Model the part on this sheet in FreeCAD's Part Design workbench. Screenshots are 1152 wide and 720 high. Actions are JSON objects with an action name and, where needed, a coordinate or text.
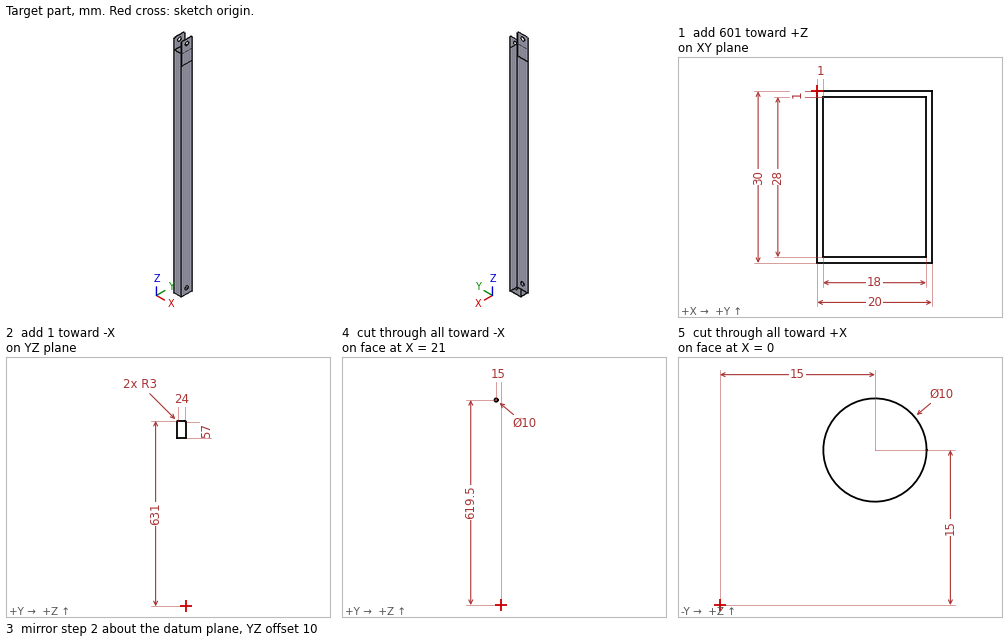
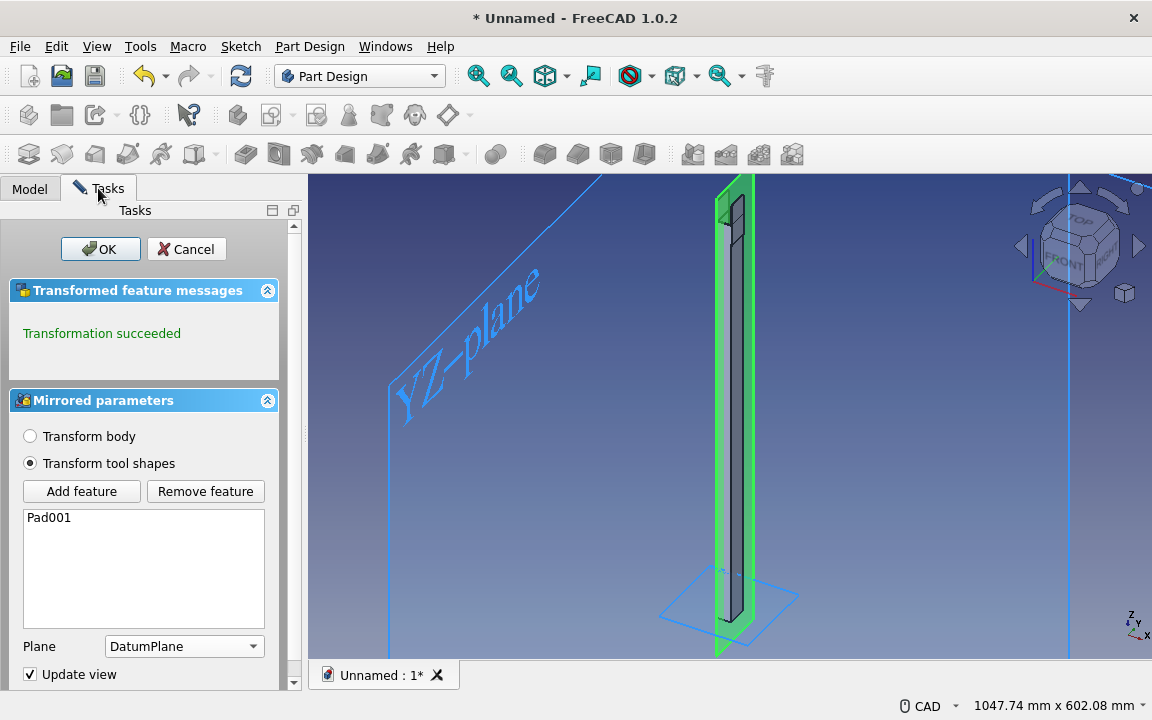
{"action": "left_click", "coordinate": [101, 249]}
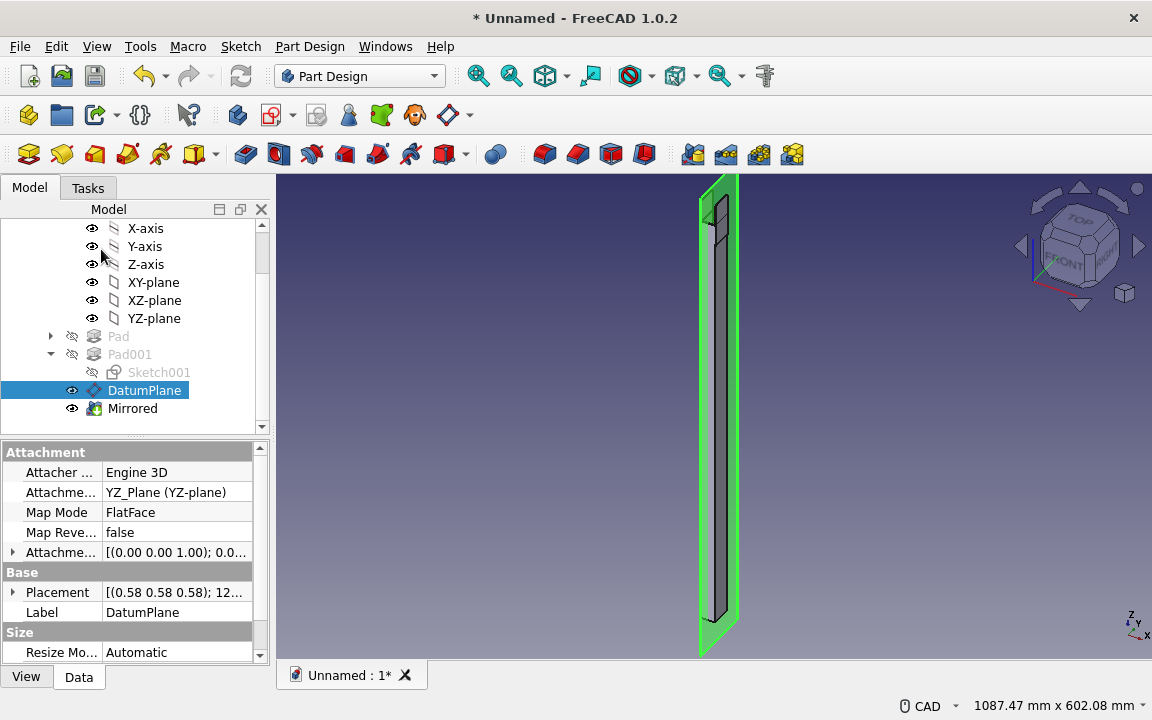
{"action": "left_click", "coordinate": [117, 390]}
{"action": "key", "text": "space"}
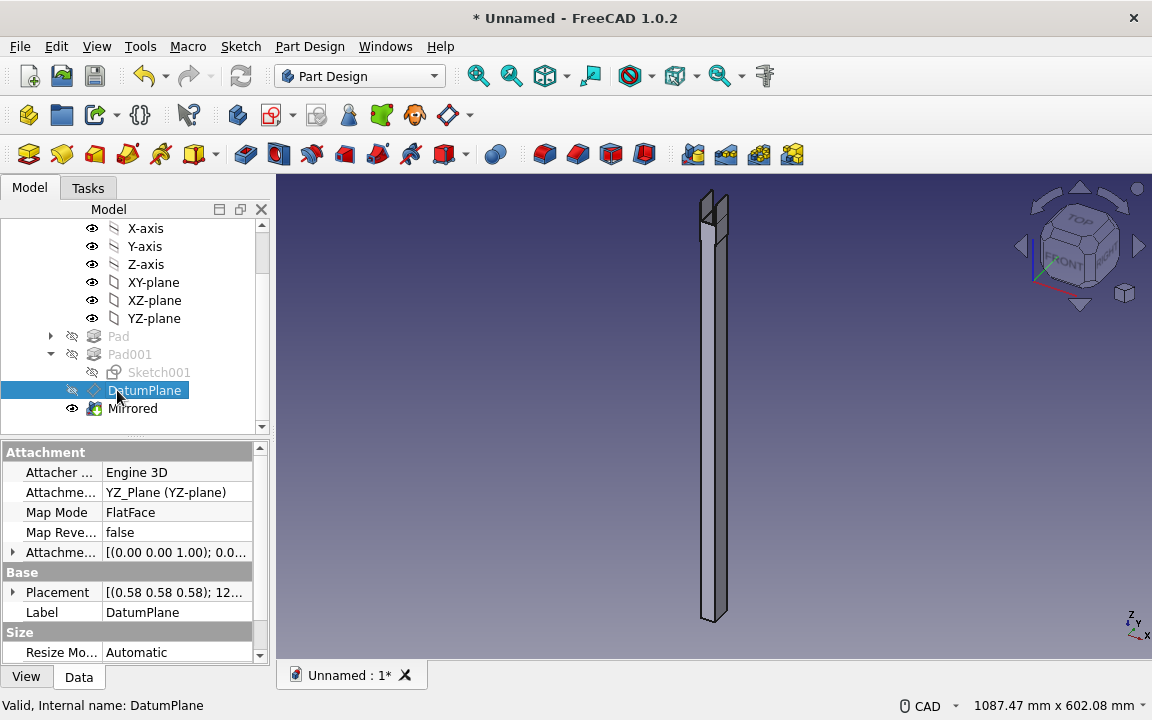
{"action": "key", "text": "0"}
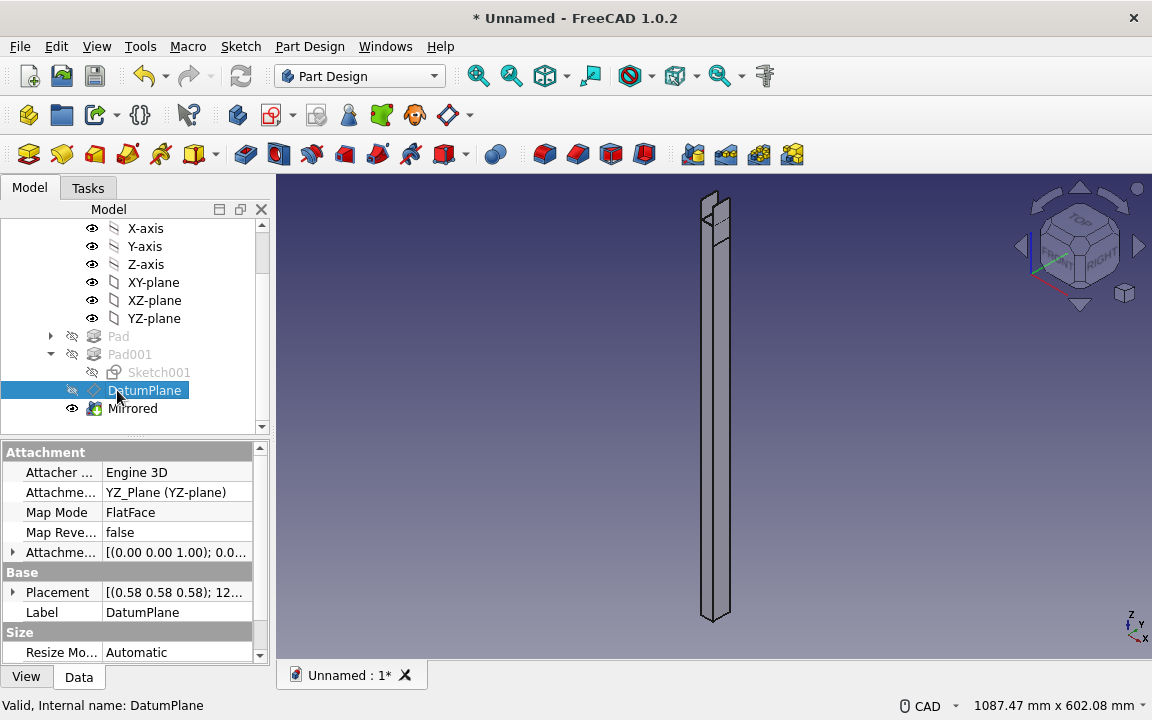
{"action": "left_click", "coordinate": [722, 215]}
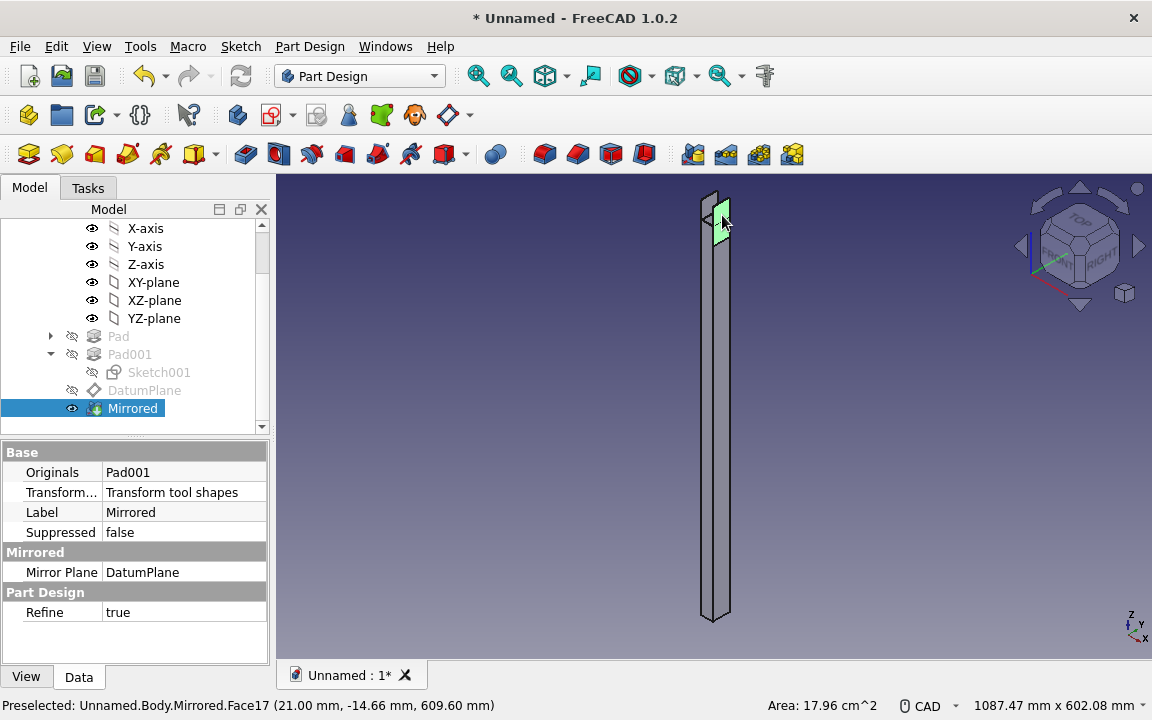
{"action": "left_click", "coordinate": [270, 116]}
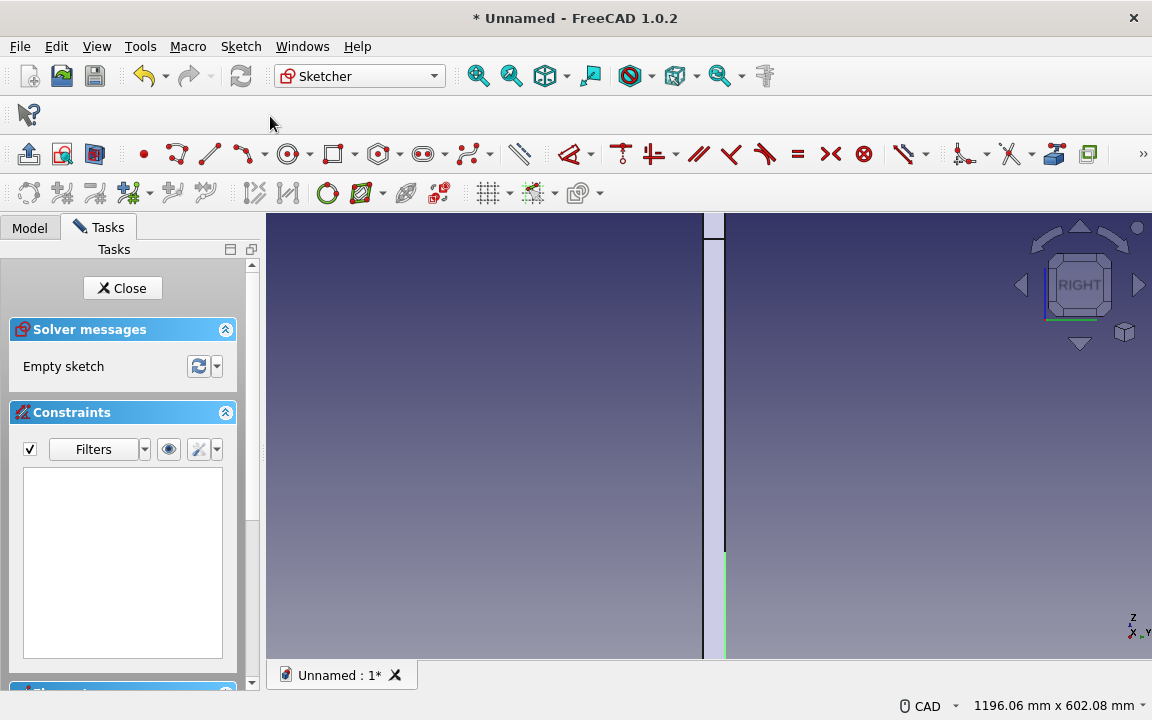
{"action": "scroll", "coordinate": [640, 436], "scroll_direction": "down", "scroll_amount": 5}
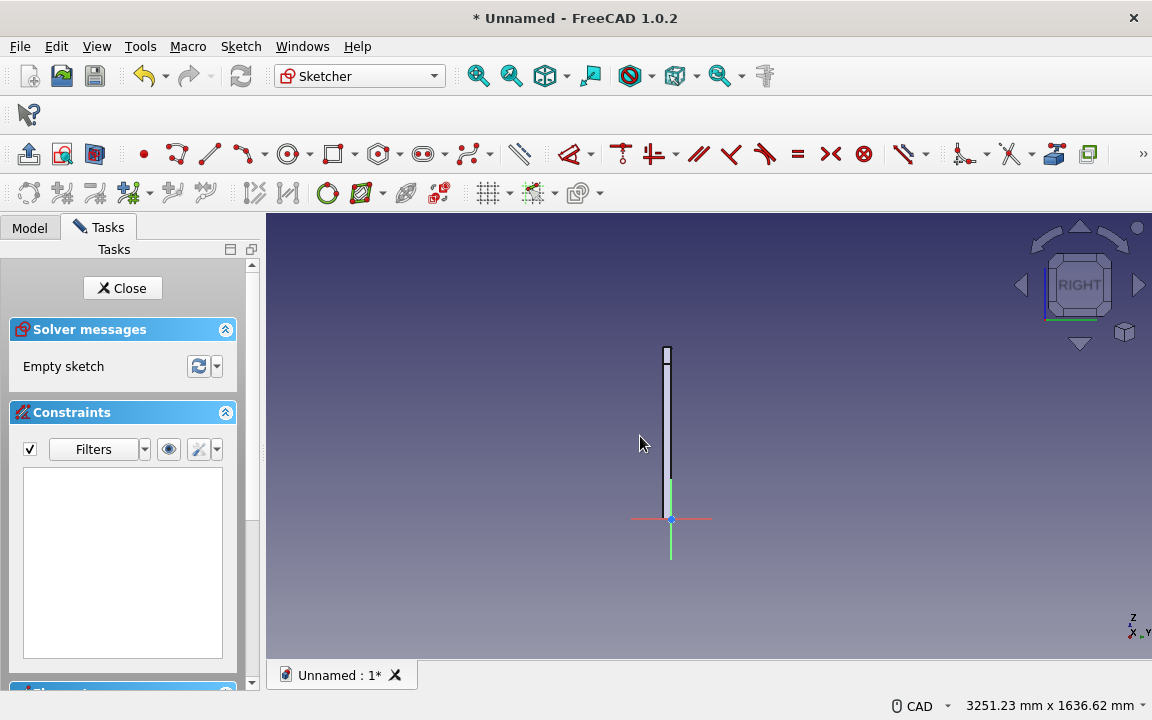
{"action": "scroll", "coordinate": [669, 346], "scroll_direction": "up", "scroll_amount": 15}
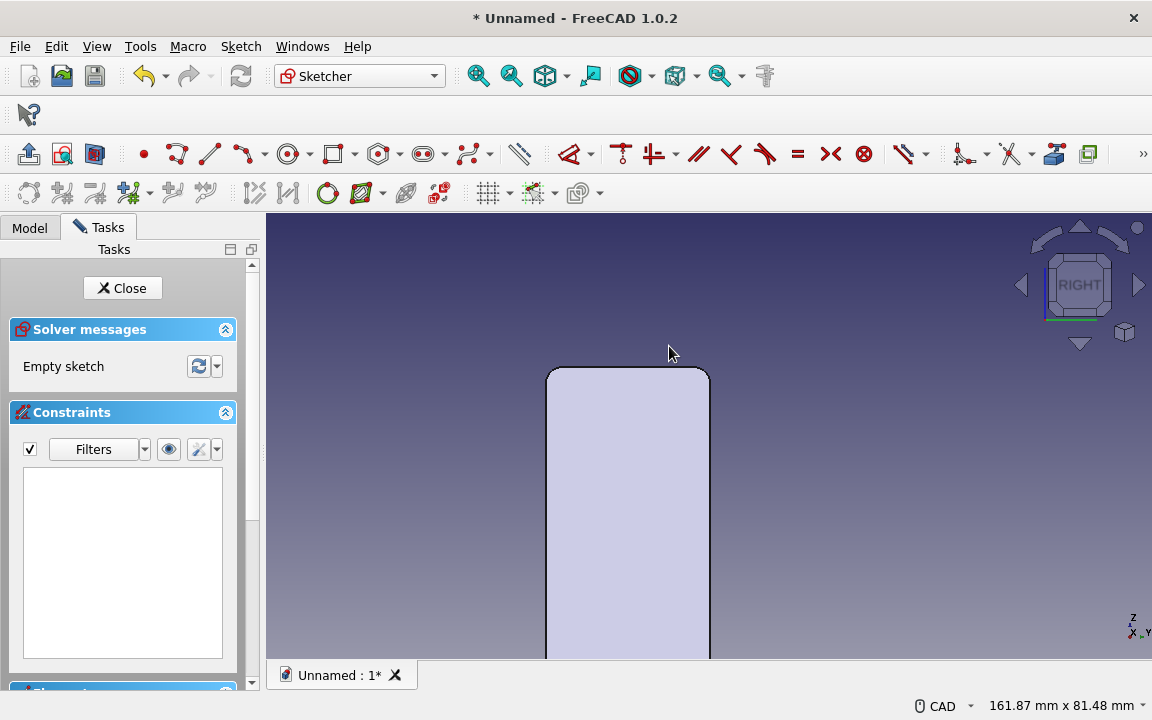
{"action": "scroll", "coordinate": [625, 429], "scroll_direction": "up", "scroll_amount": 8}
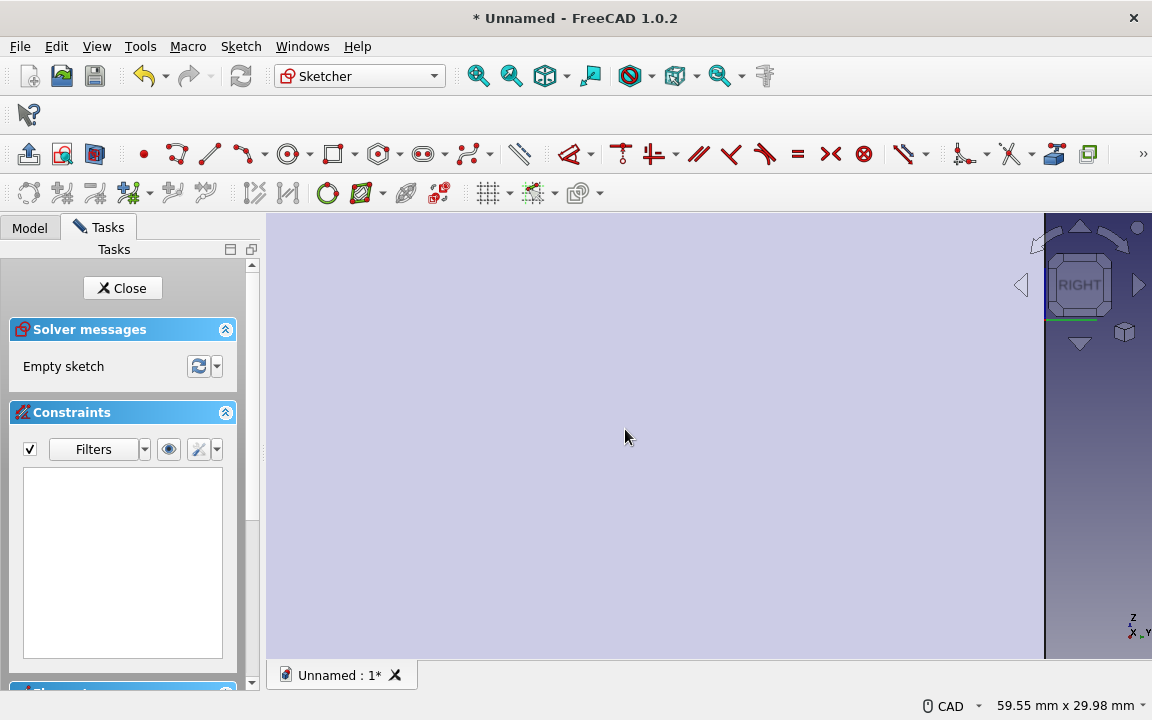
{"action": "key", "text": "g c"}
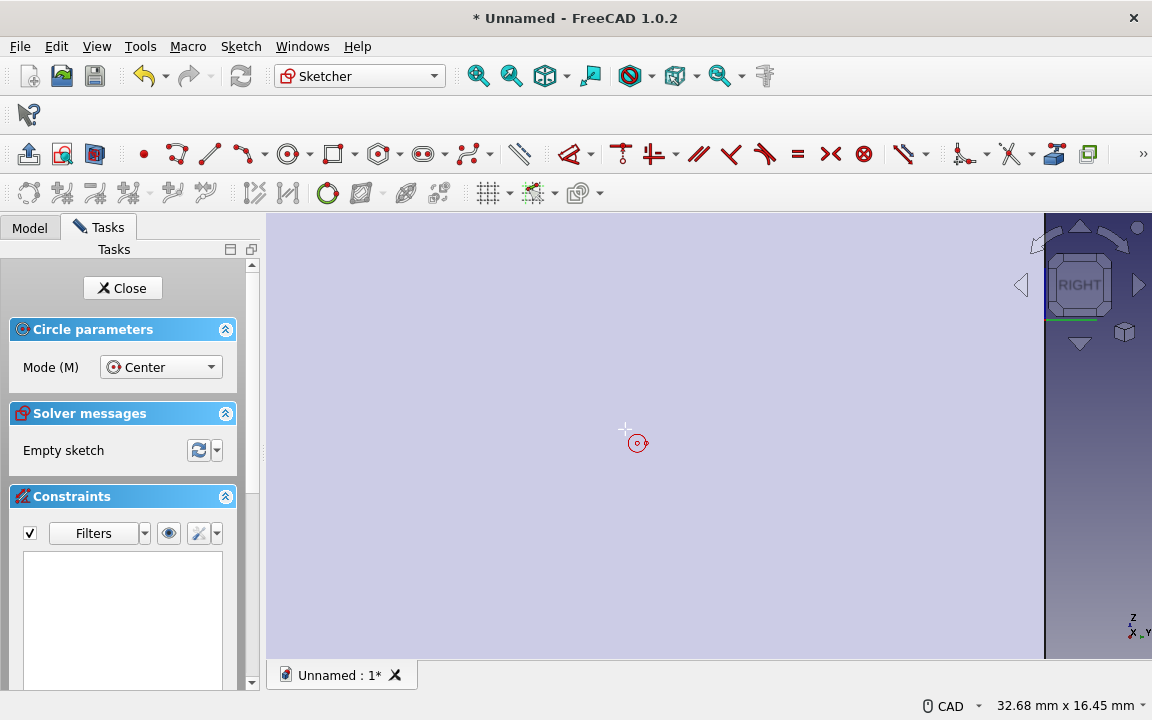
{"action": "left_click", "coordinate": [638, 432]}
{"action": "left_click", "coordinate": [734, 336]}
{"action": "key", "text": "Escape"}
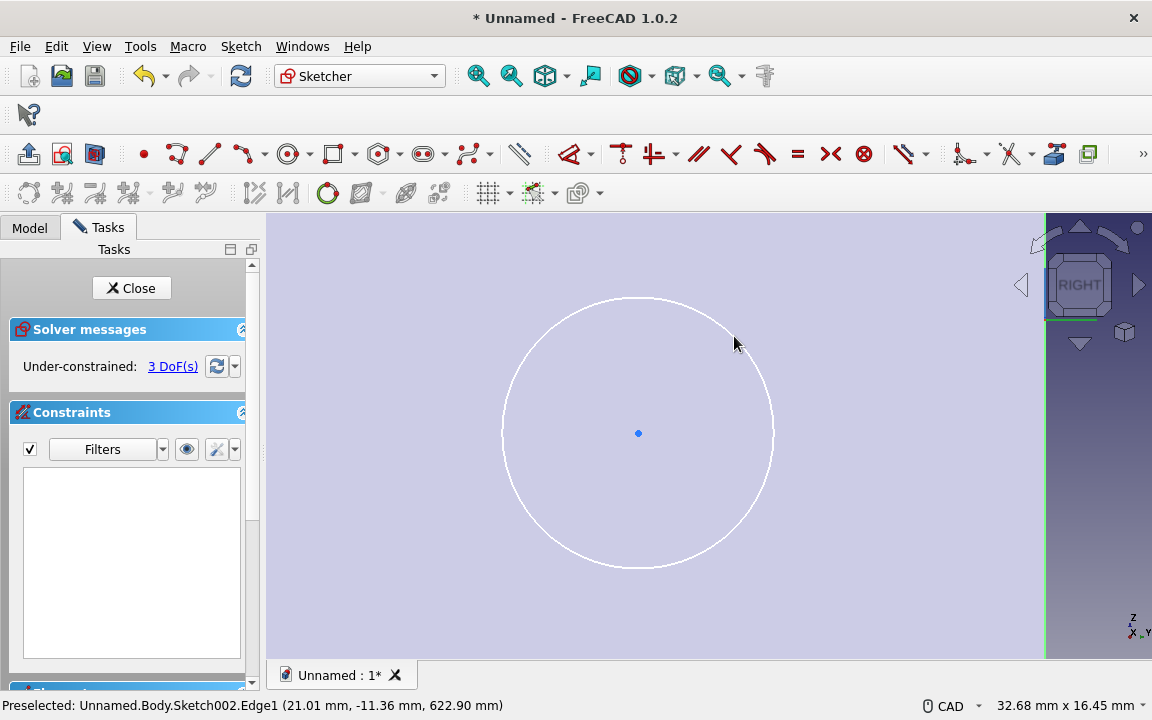
{"action": "left_click", "coordinate": [568, 154]}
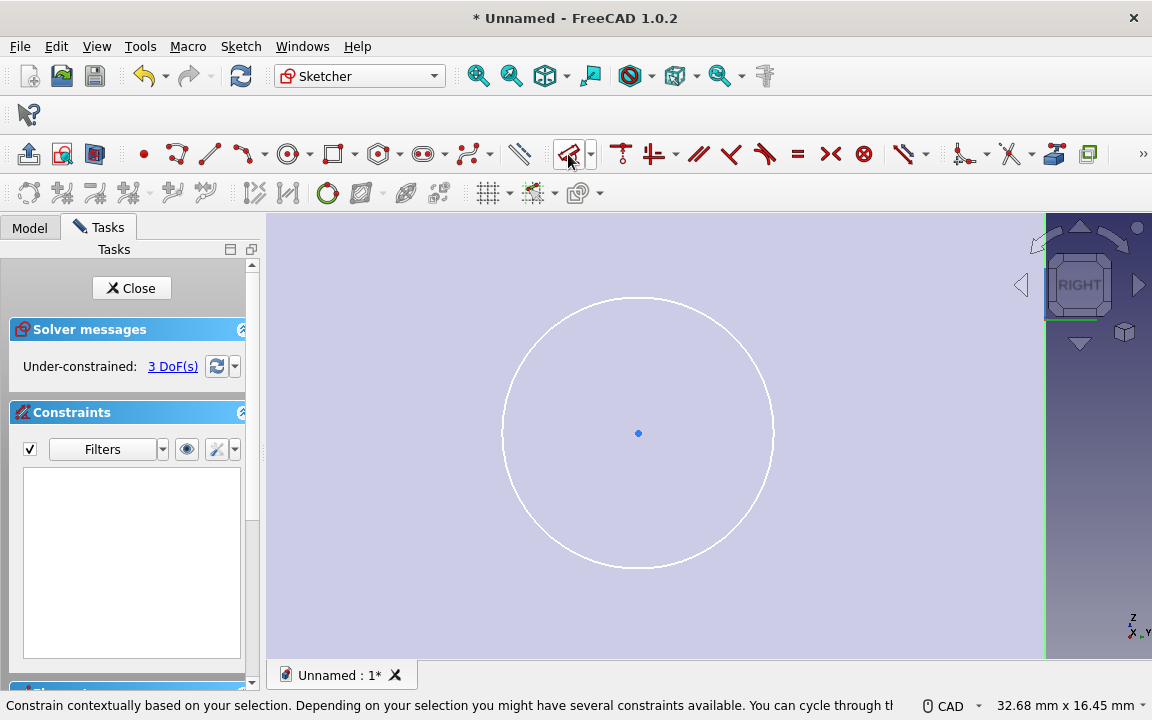
{"action": "left_click", "coordinate": [734, 337]}
{"action": "left_click", "coordinate": [757, 314]}